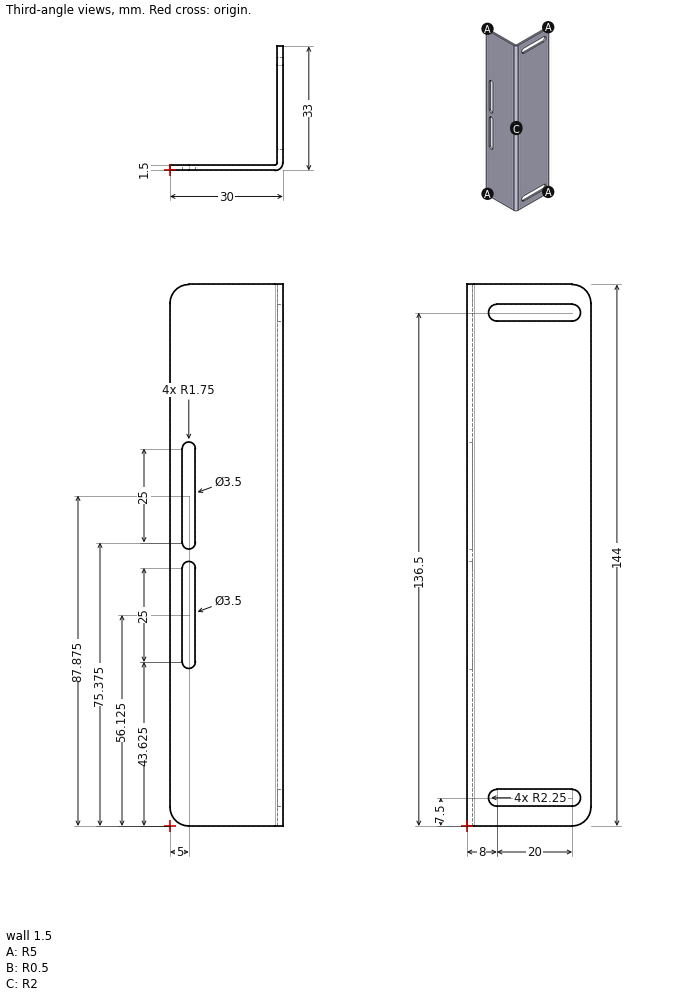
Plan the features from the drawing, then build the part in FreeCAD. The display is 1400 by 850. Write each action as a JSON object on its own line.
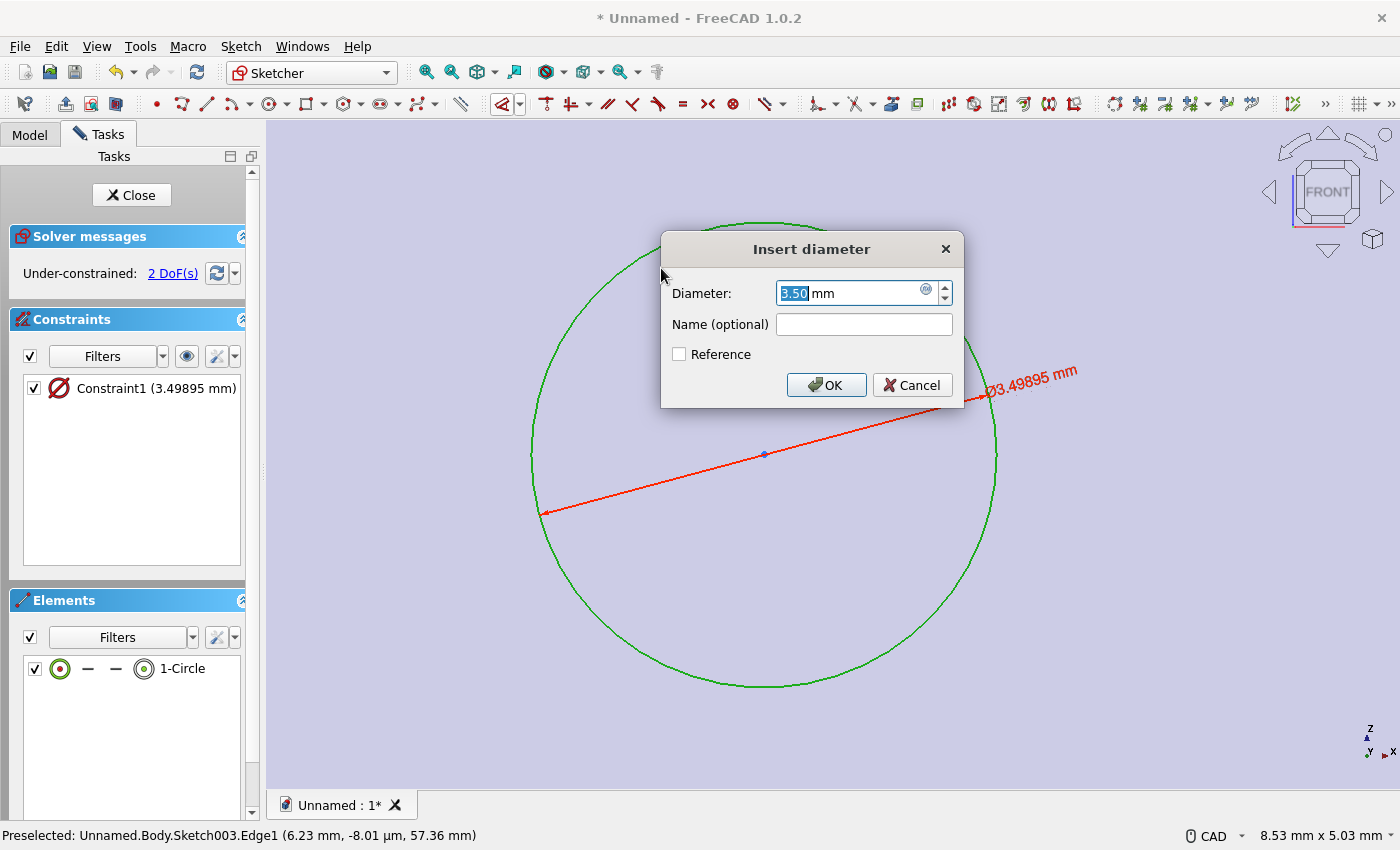
{"action": "type", "text": "3.5"}
{"action": "key", "text": "Return"}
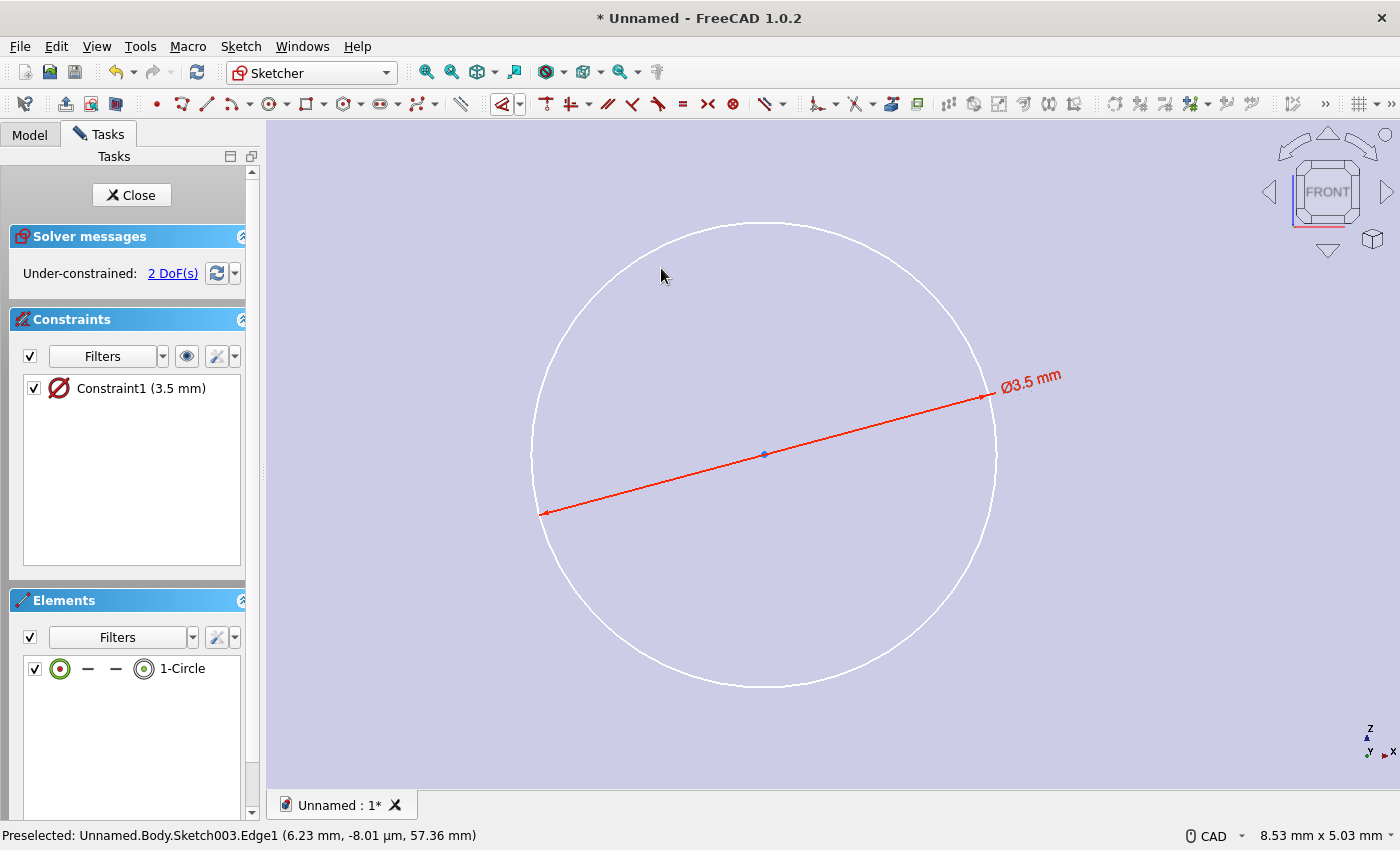
{"action": "left_click", "coordinate": [764, 455]}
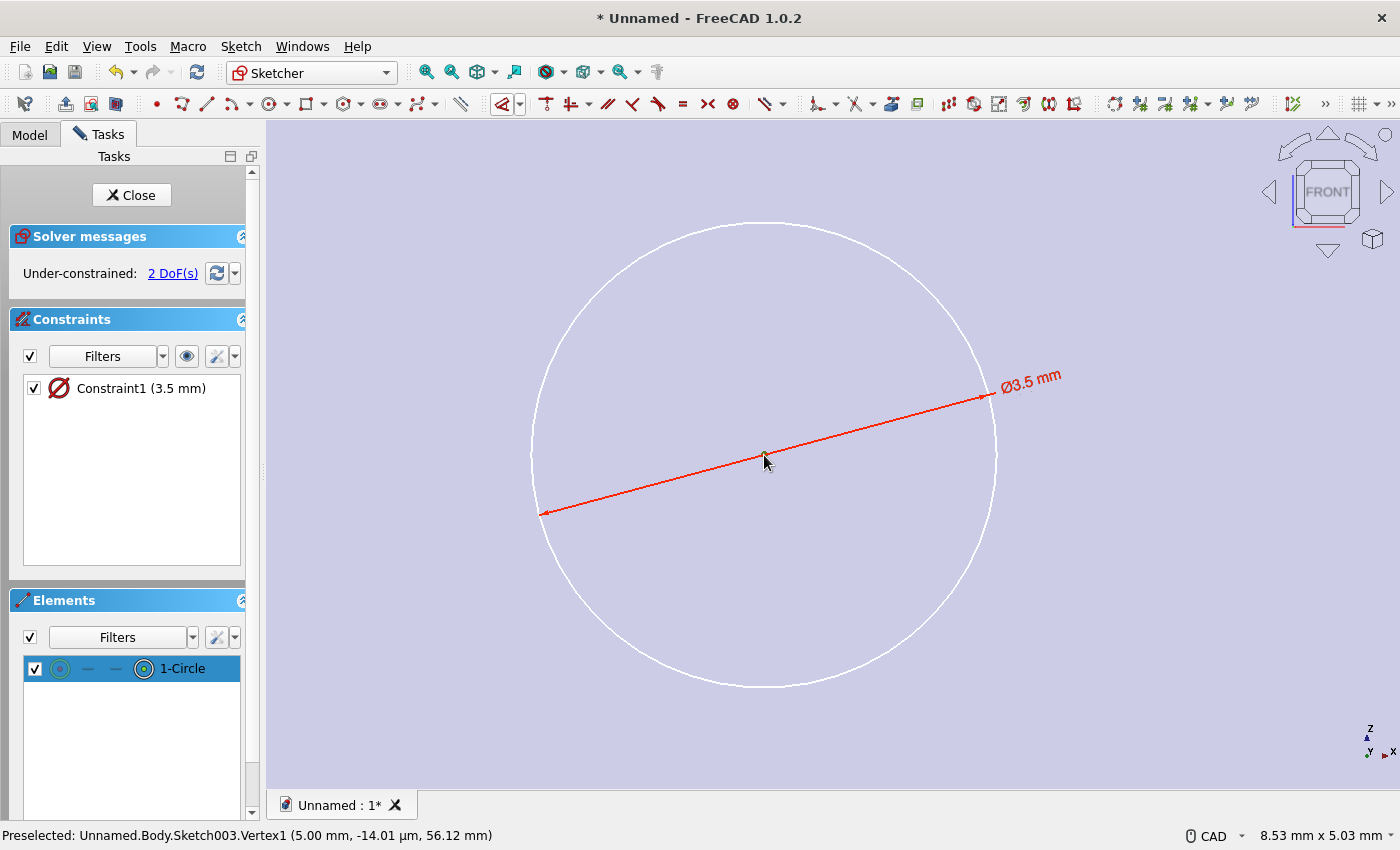
{"action": "key", "text": "l"}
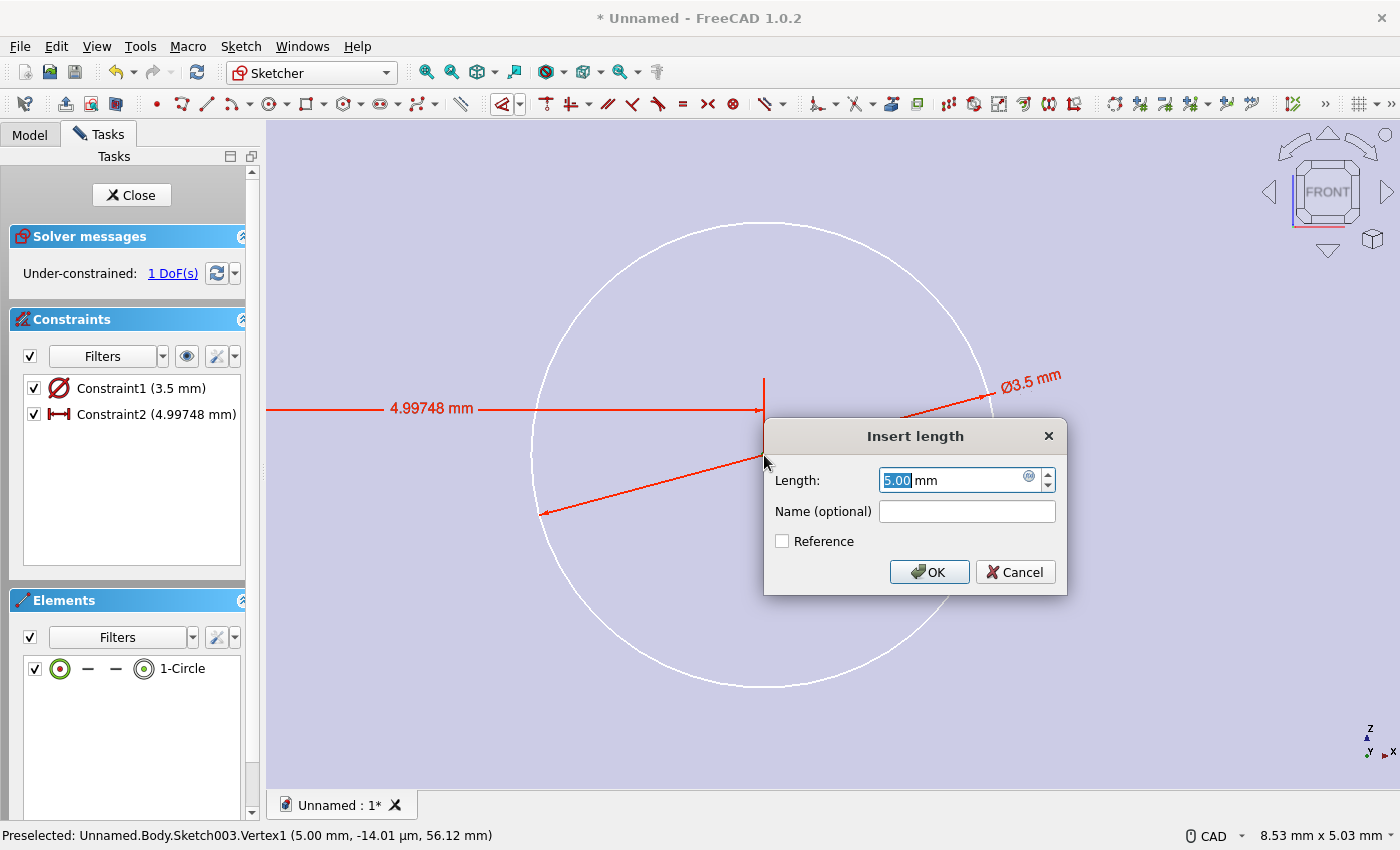
{"action": "type", "text": "5"}
{"action": "key", "text": "Return"}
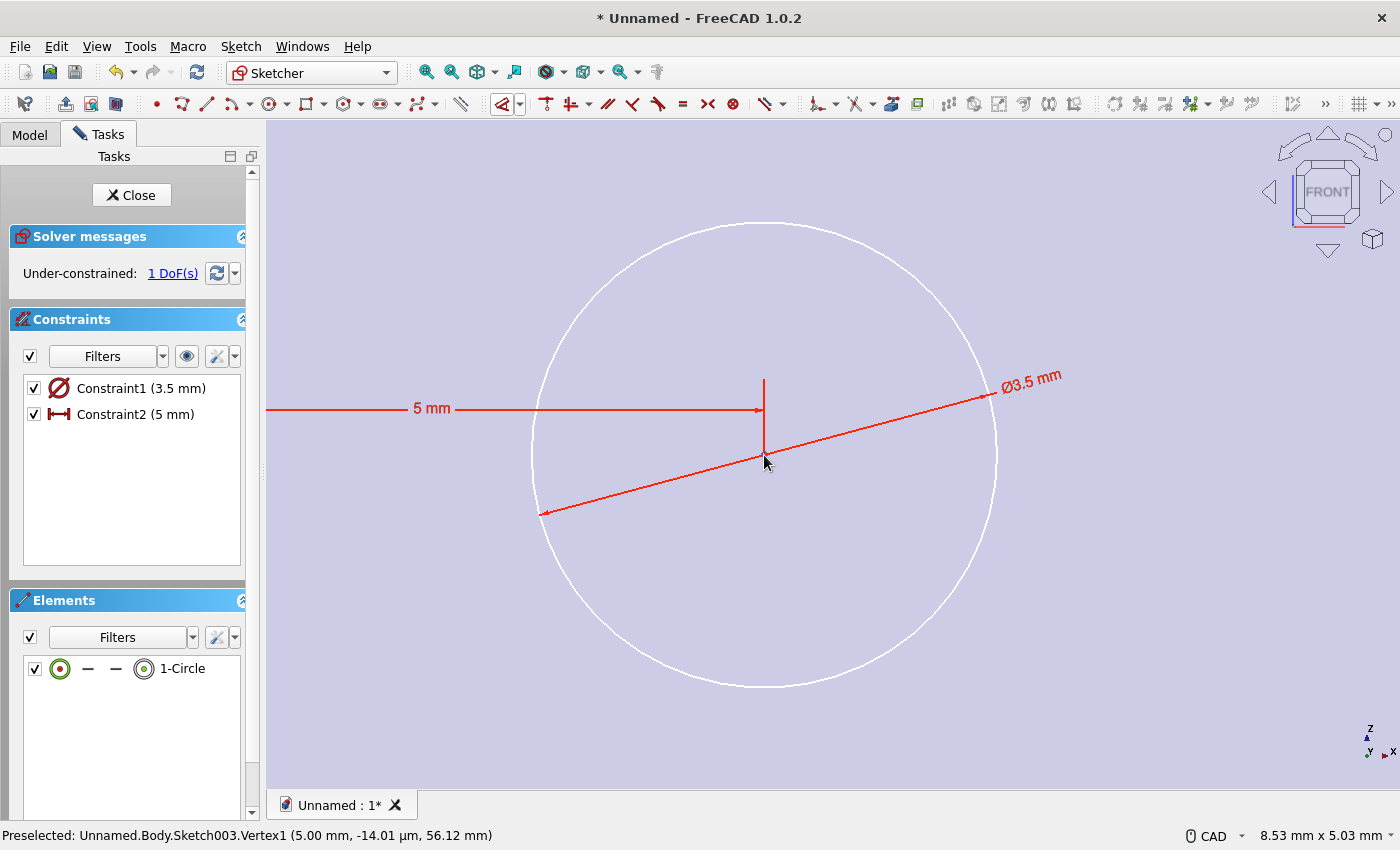
{"action": "left_click", "coordinate": [764, 455]}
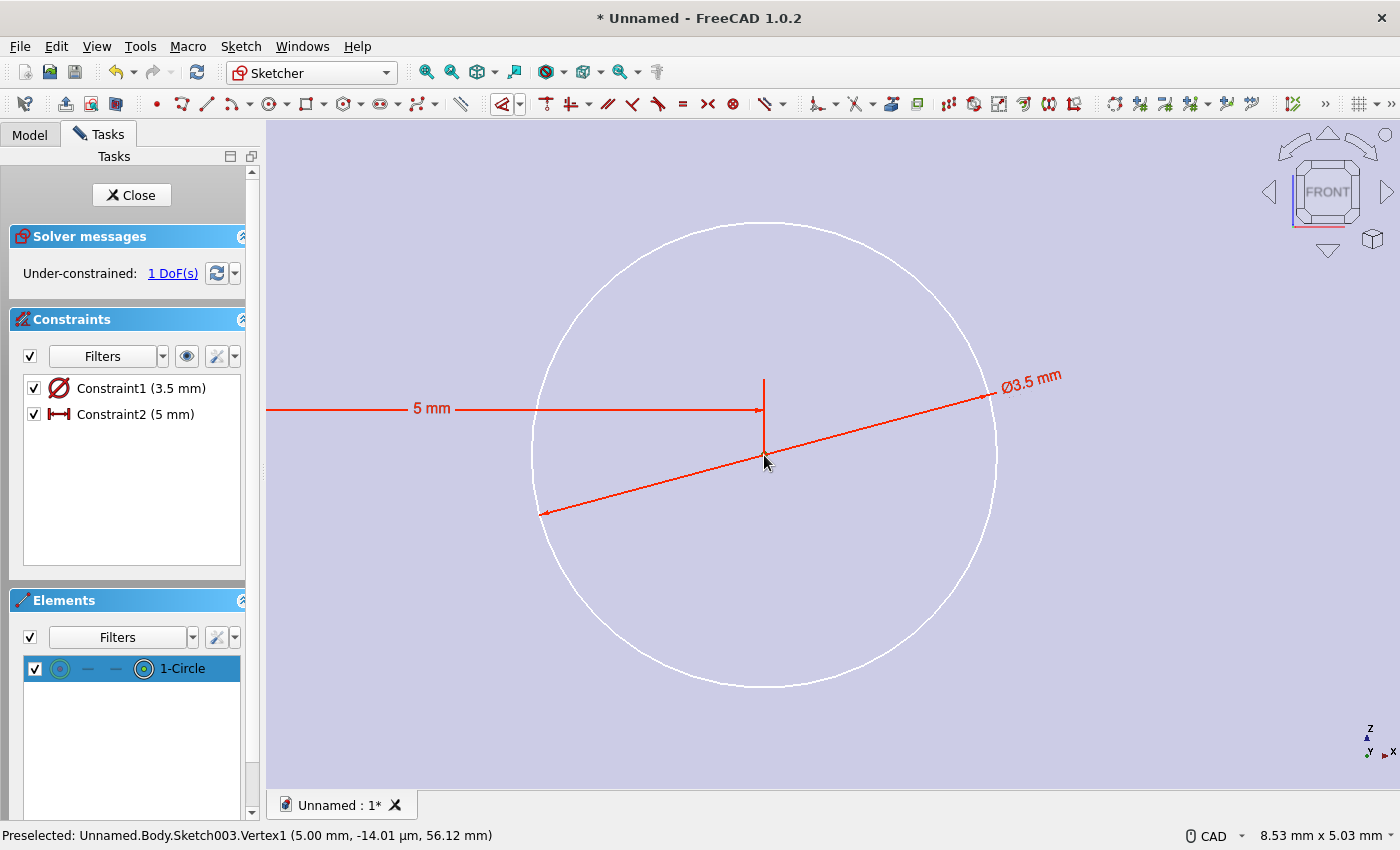
{"action": "left_click", "coordinate": [520, 104]}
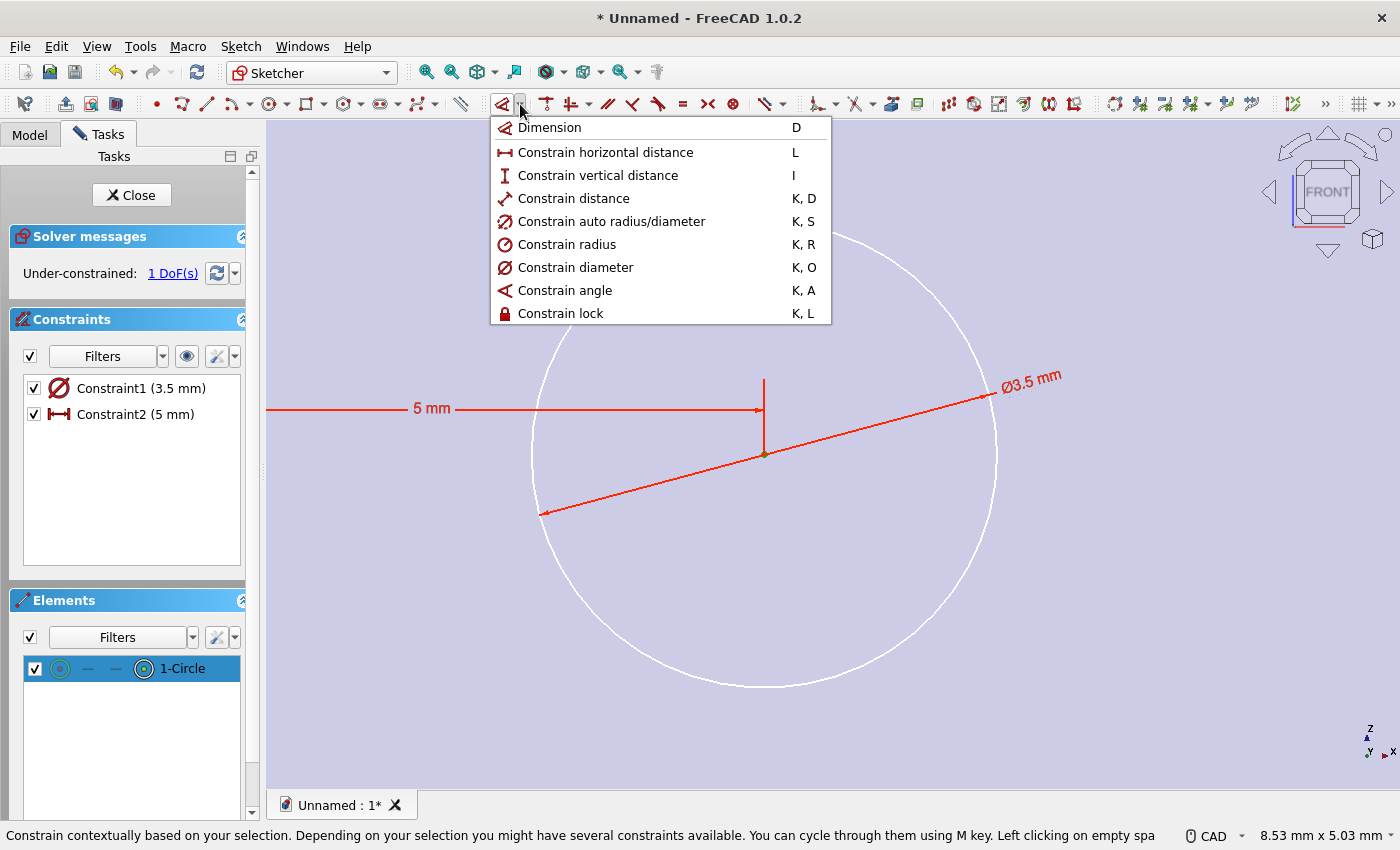
{"action": "left_click", "coordinate": [661, 176]}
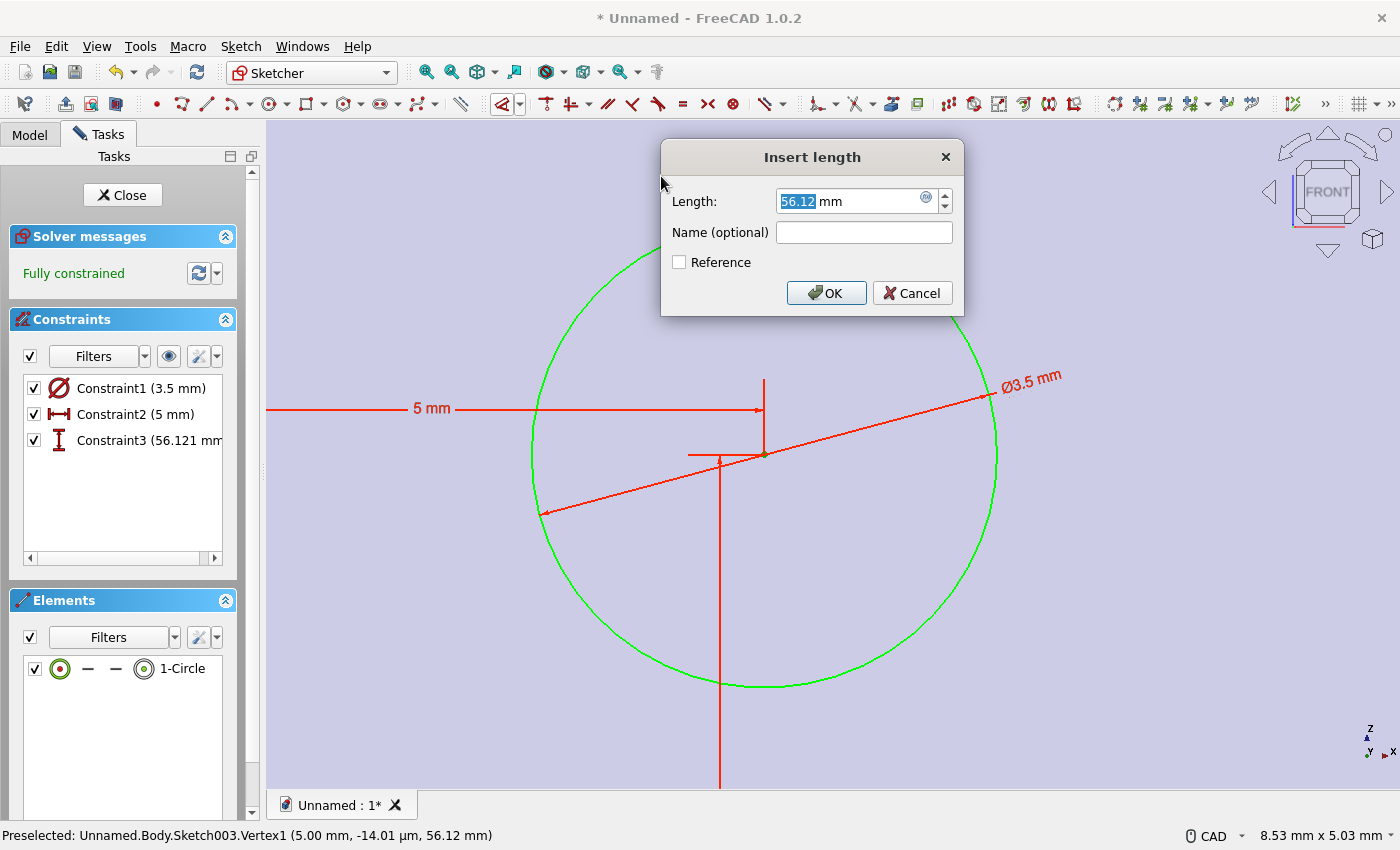
{"action": "type", "text": "56.125"}
{"action": "key", "text": "Return"}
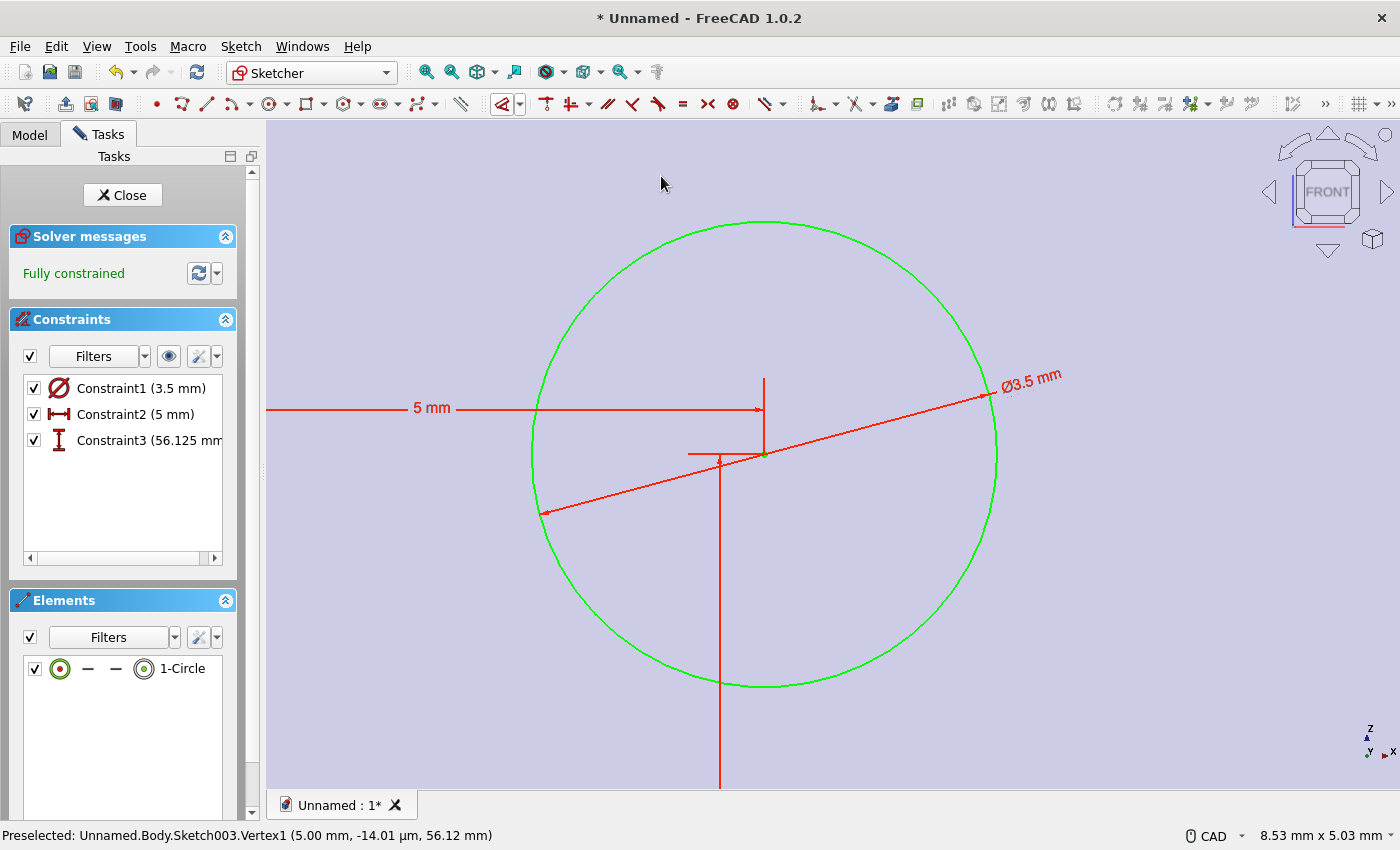
{"action": "left_click", "coordinate": [123, 195]}